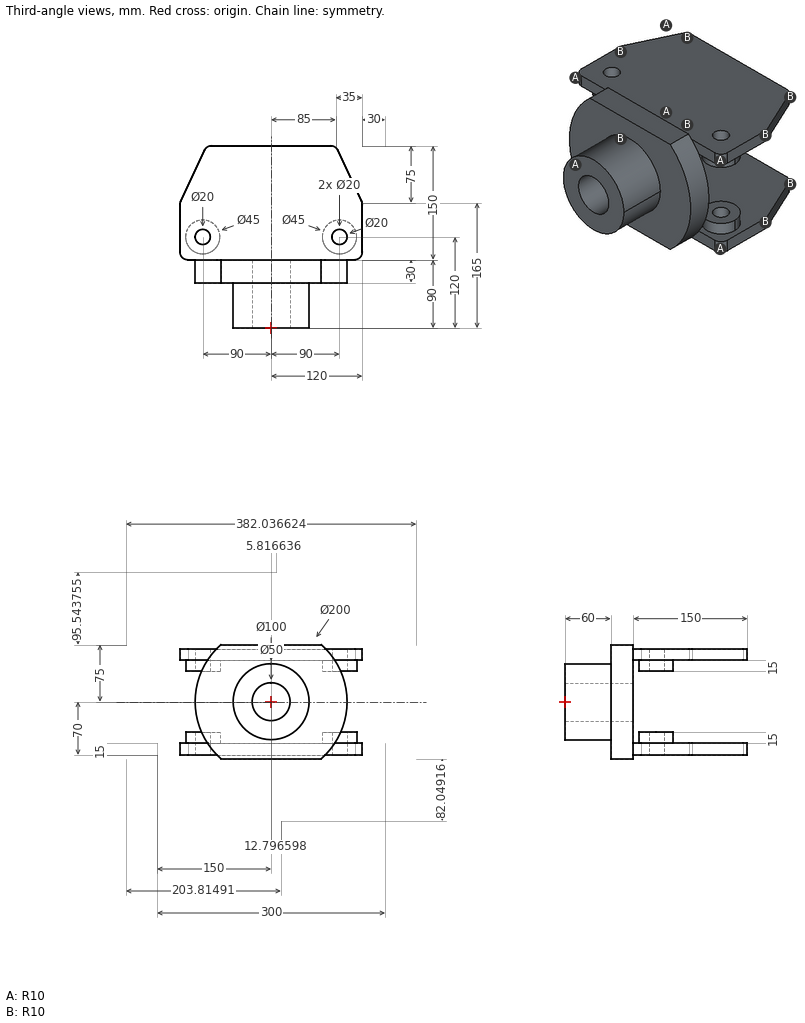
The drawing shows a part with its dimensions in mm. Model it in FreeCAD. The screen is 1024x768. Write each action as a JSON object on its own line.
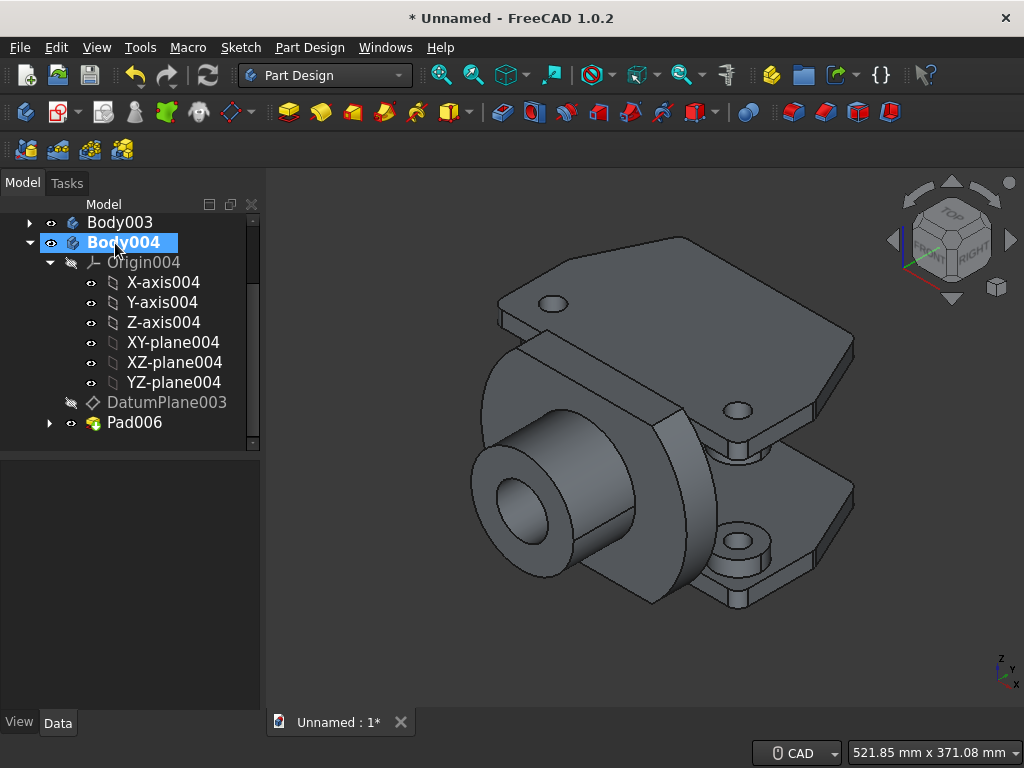
{"action": "key", "text": "v f"}